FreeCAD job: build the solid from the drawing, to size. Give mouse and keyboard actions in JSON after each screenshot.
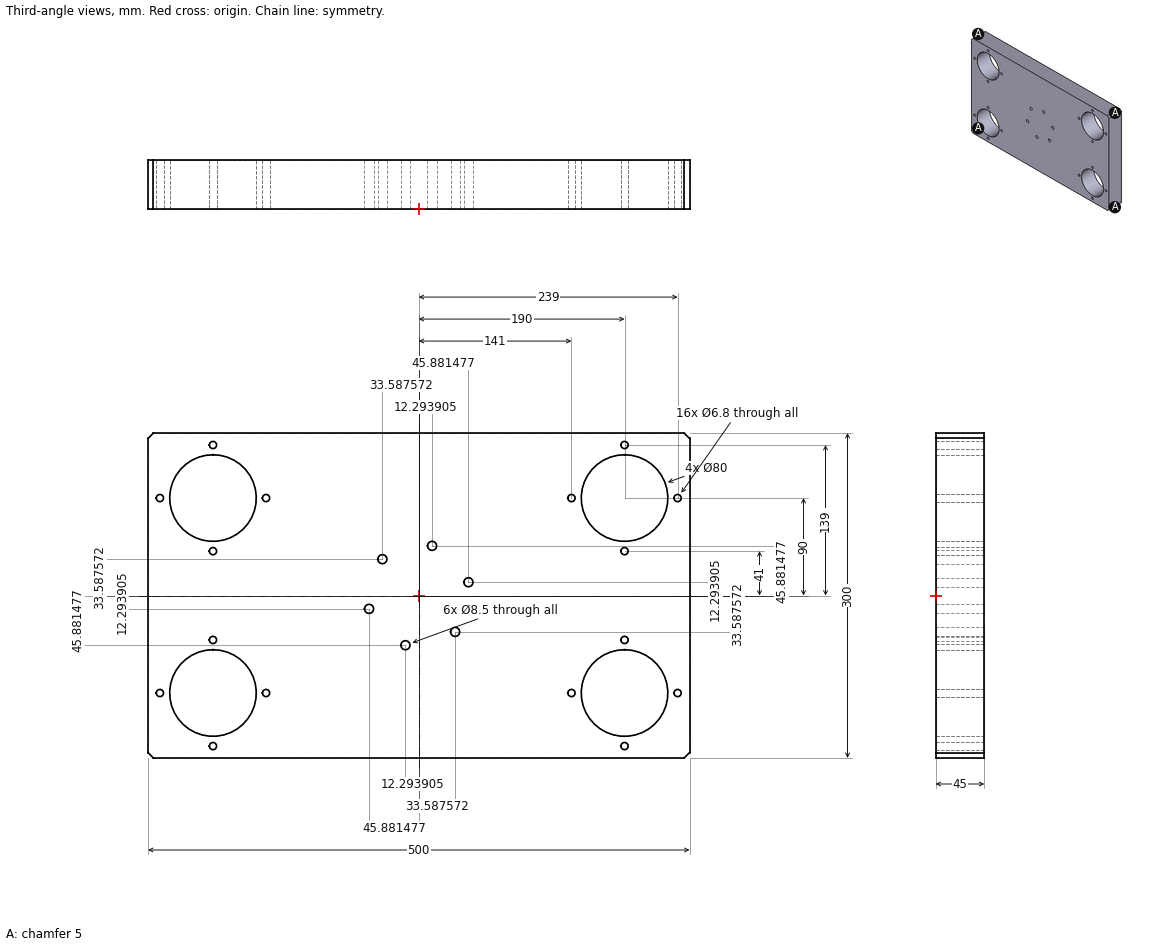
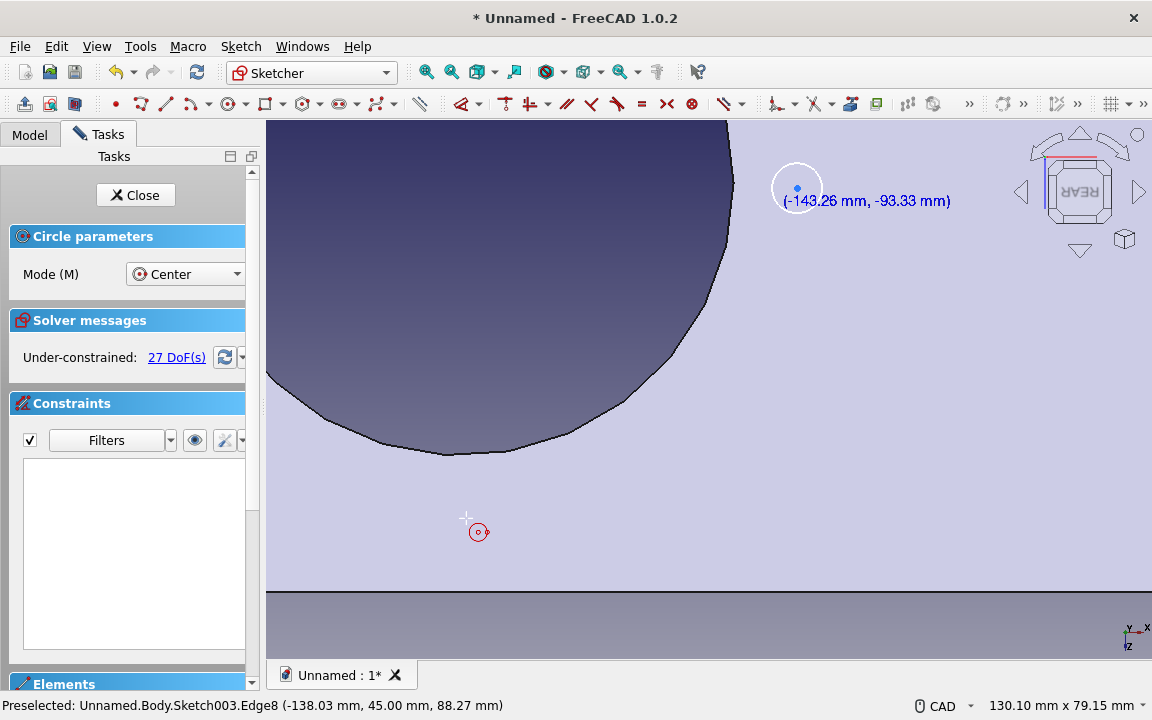
{"action": "scroll", "coordinate": [466, 518], "scroll_direction": "down", "scroll_amount": 10}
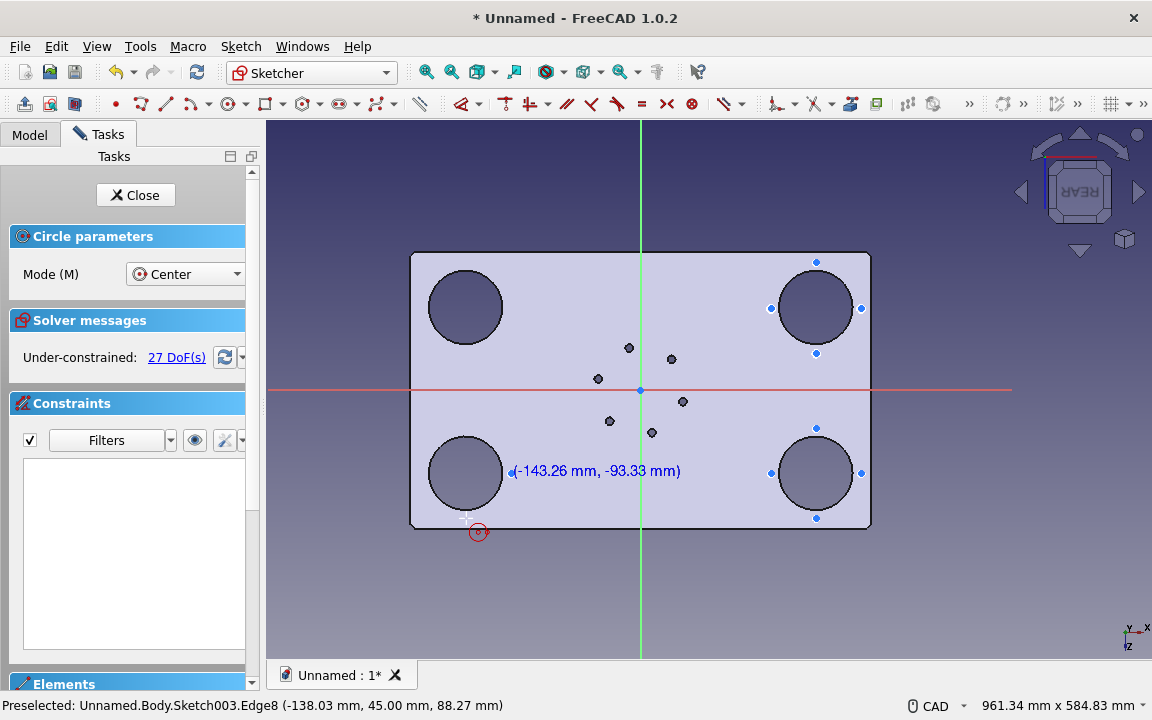
{"action": "left_click", "coordinate": [466, 518]}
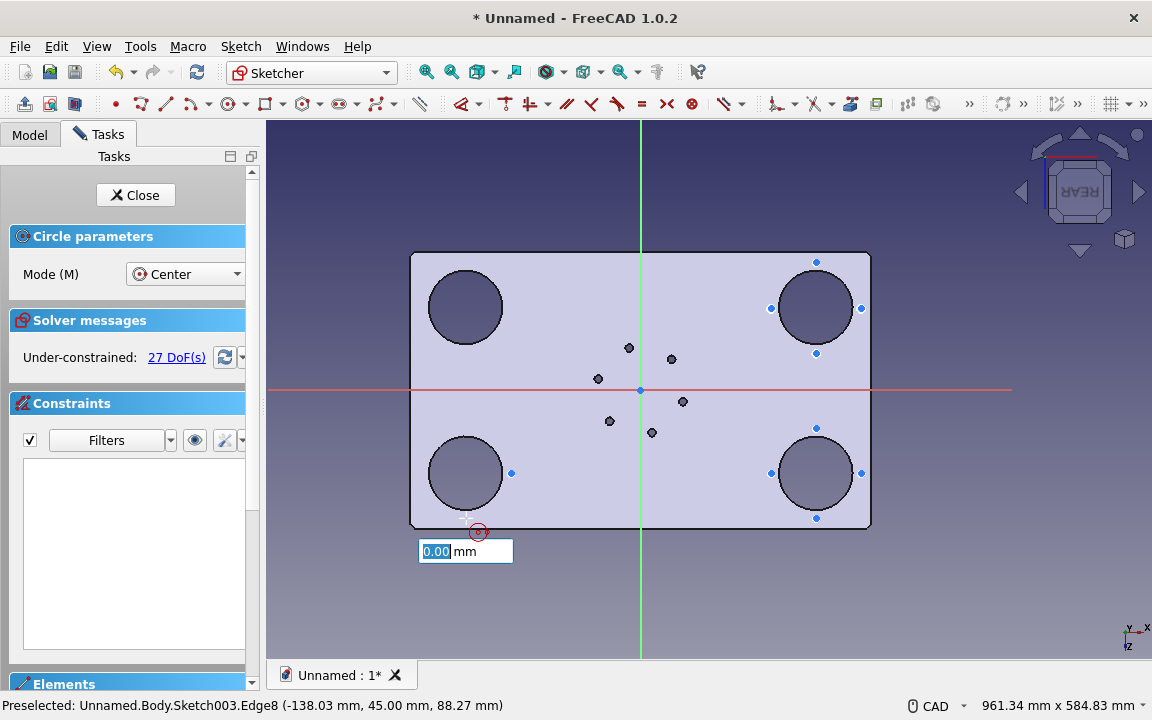
{"action": "scroll", "coordinate": [468, 516], "scroll_direction": "up", "scroll_amount": 9}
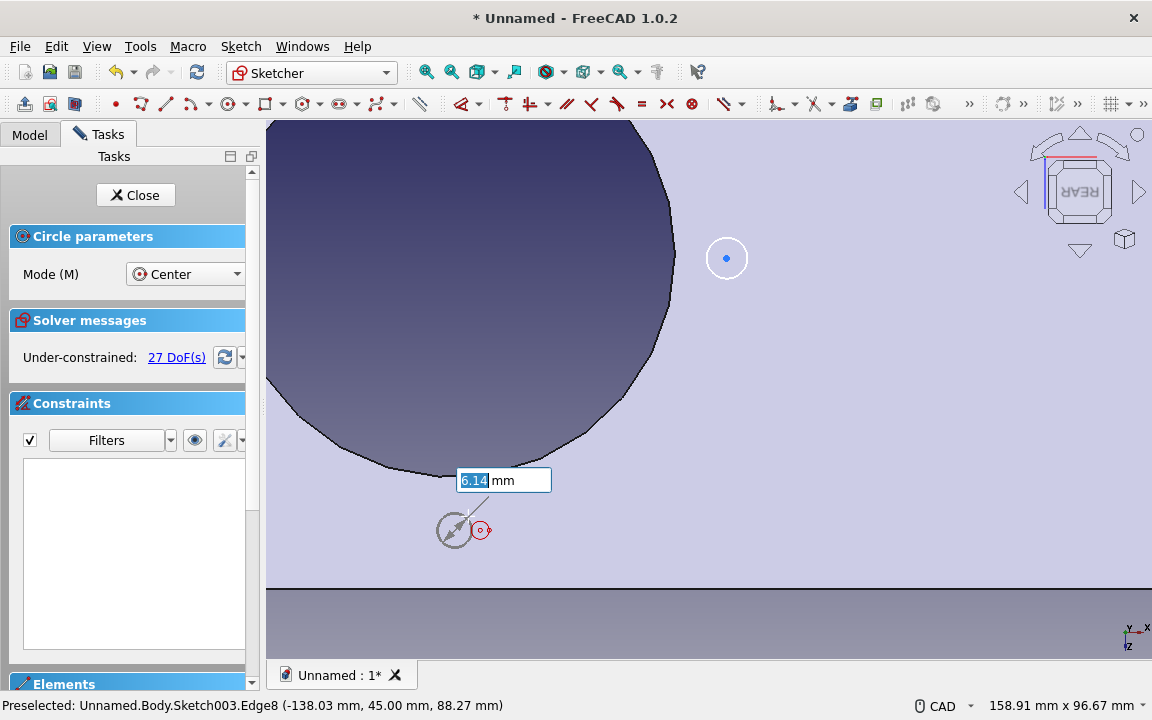
{"action": "left_click", "coordinate": [465, 514]}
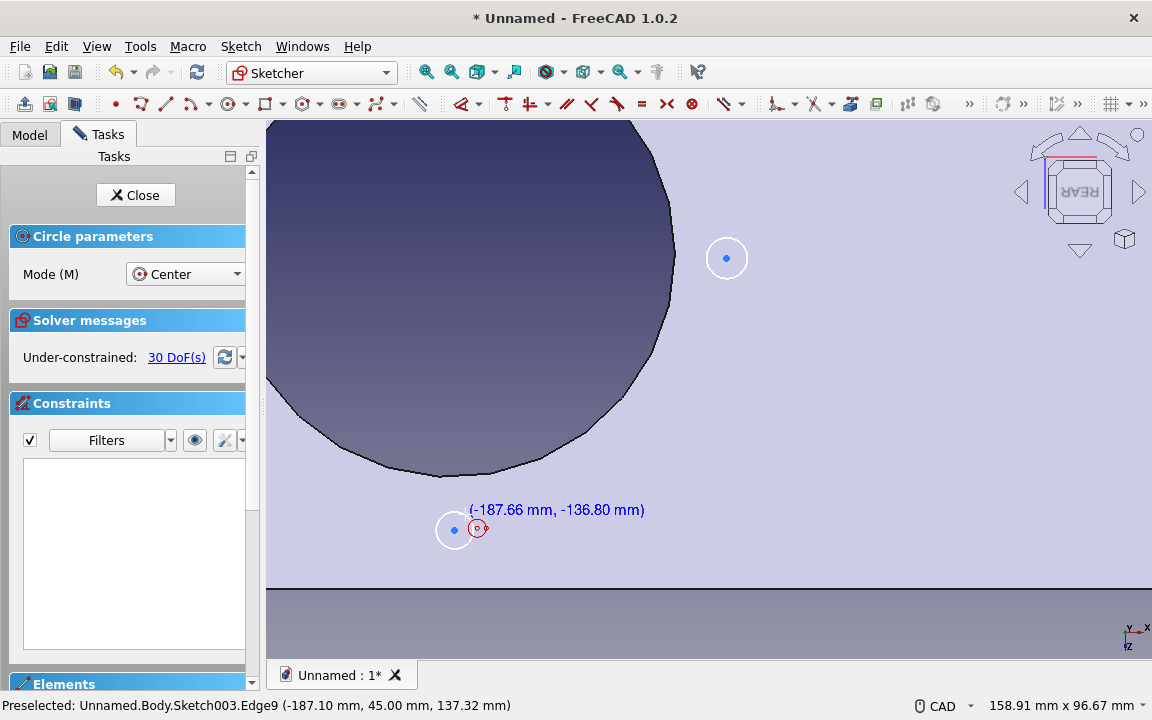
{"action": "scroll", "coordinate": [468, 516], "scroll_direction": "down", "scroll_amount": 9}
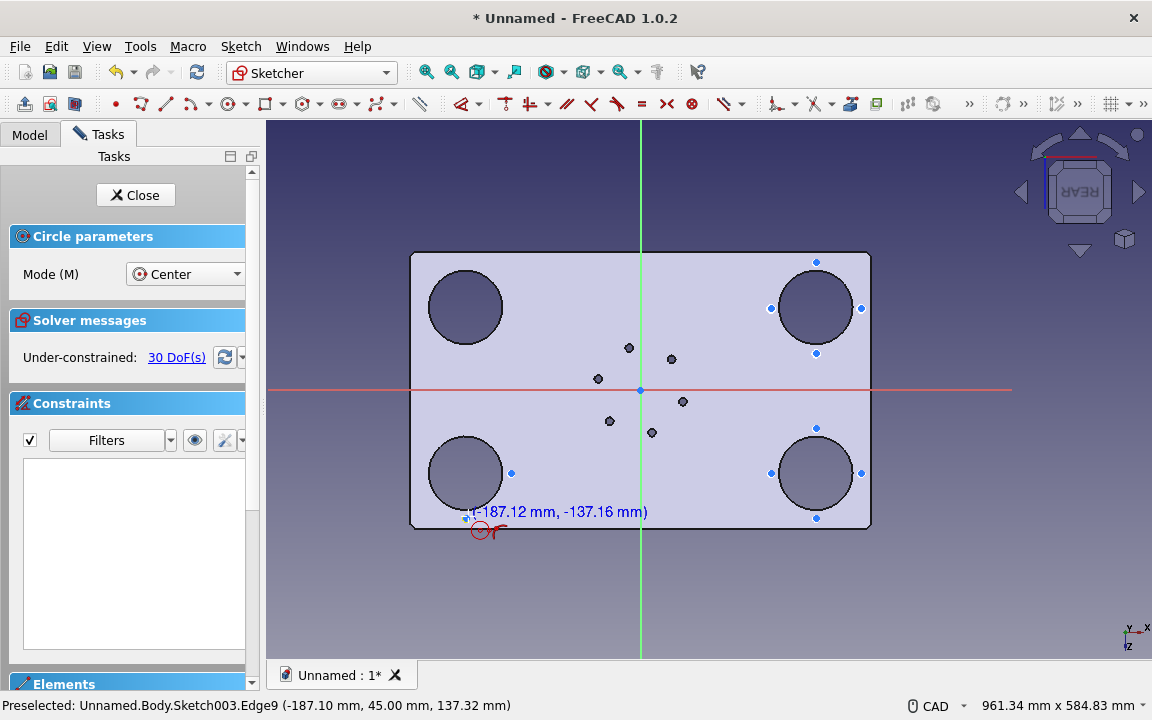
{"action": "scroll", "coordinate": [420, 473], "scroll_direction": "up", "scroll_amount": 10}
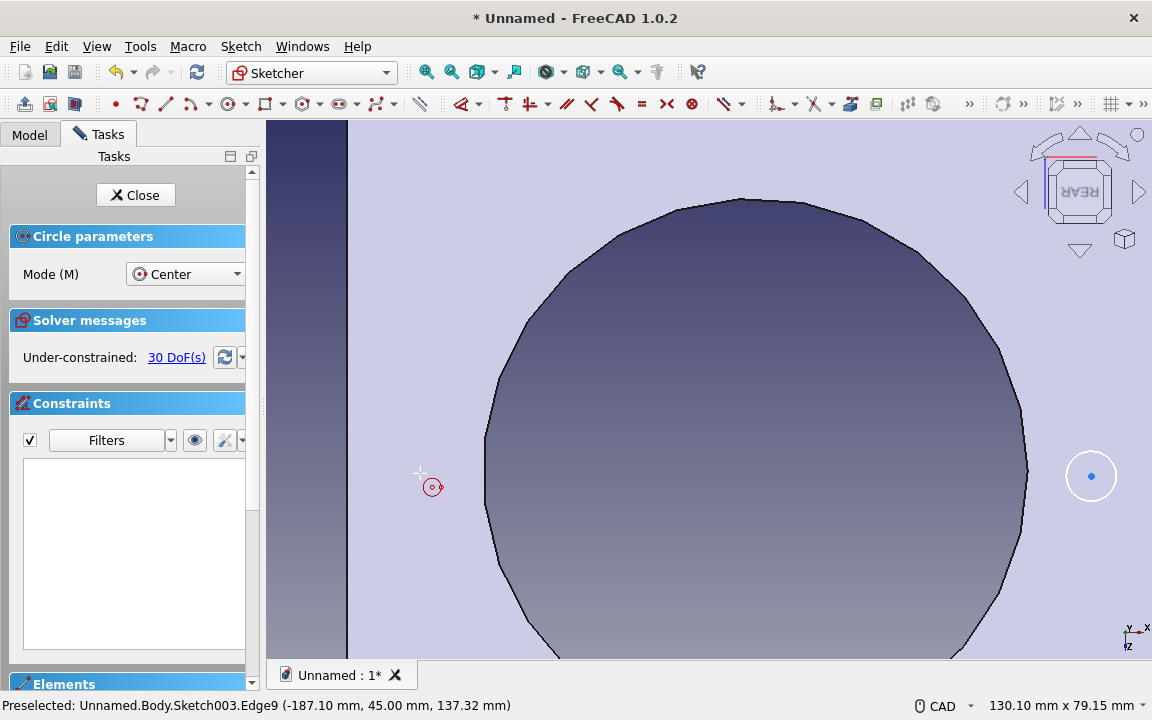
{"action": "scroll", "coordinate": [420, 473], "scroll_direction": "down", "scroll_amount": 10}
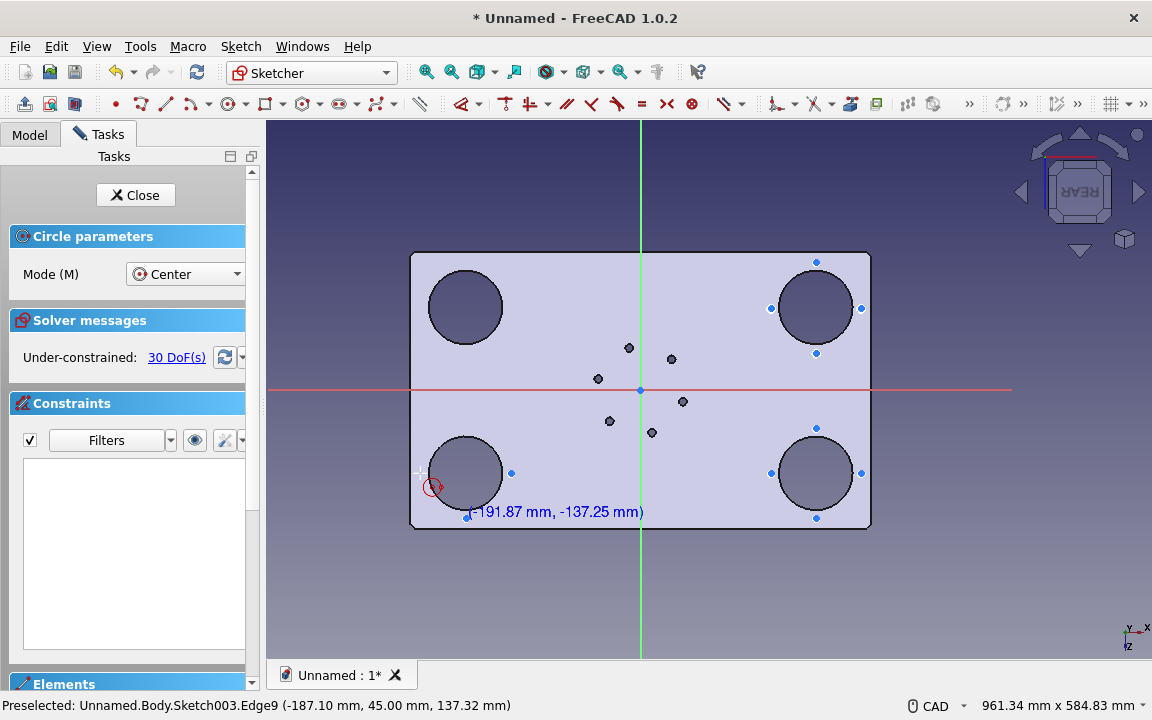
{"action": "left_click", "coordinate": [420, 473]}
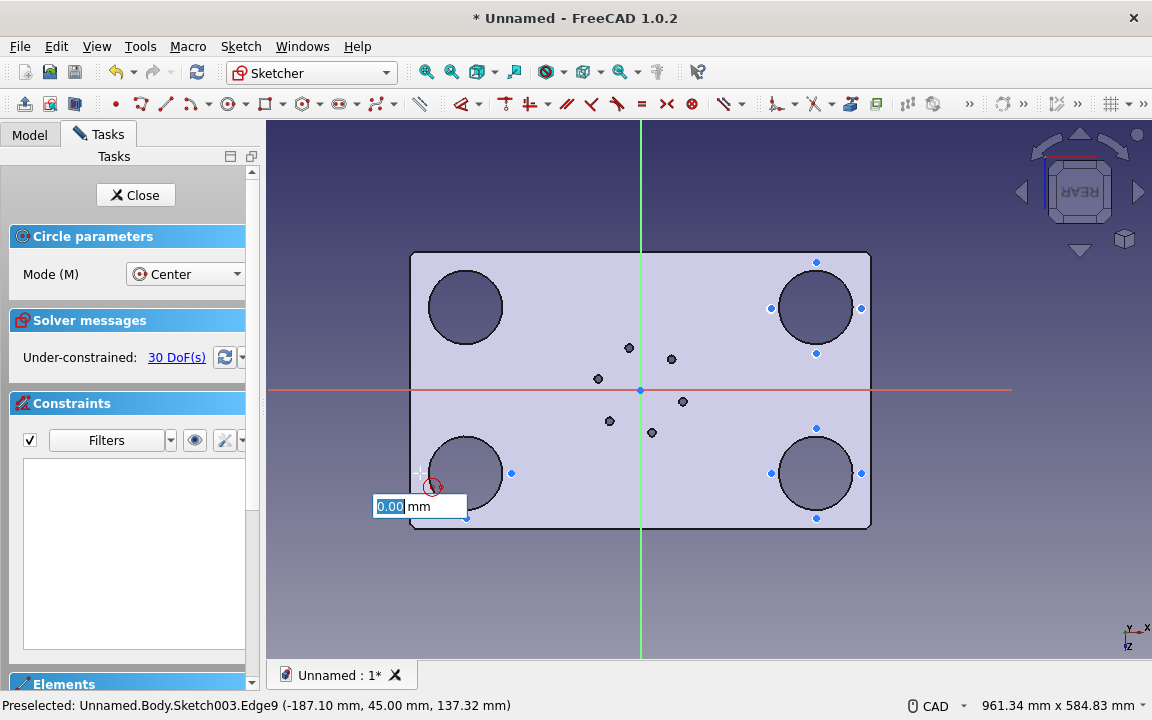
{"action": "scroll", "coordinate": [423, 471], "scroll_direction": "up", "scroll_amount": 9}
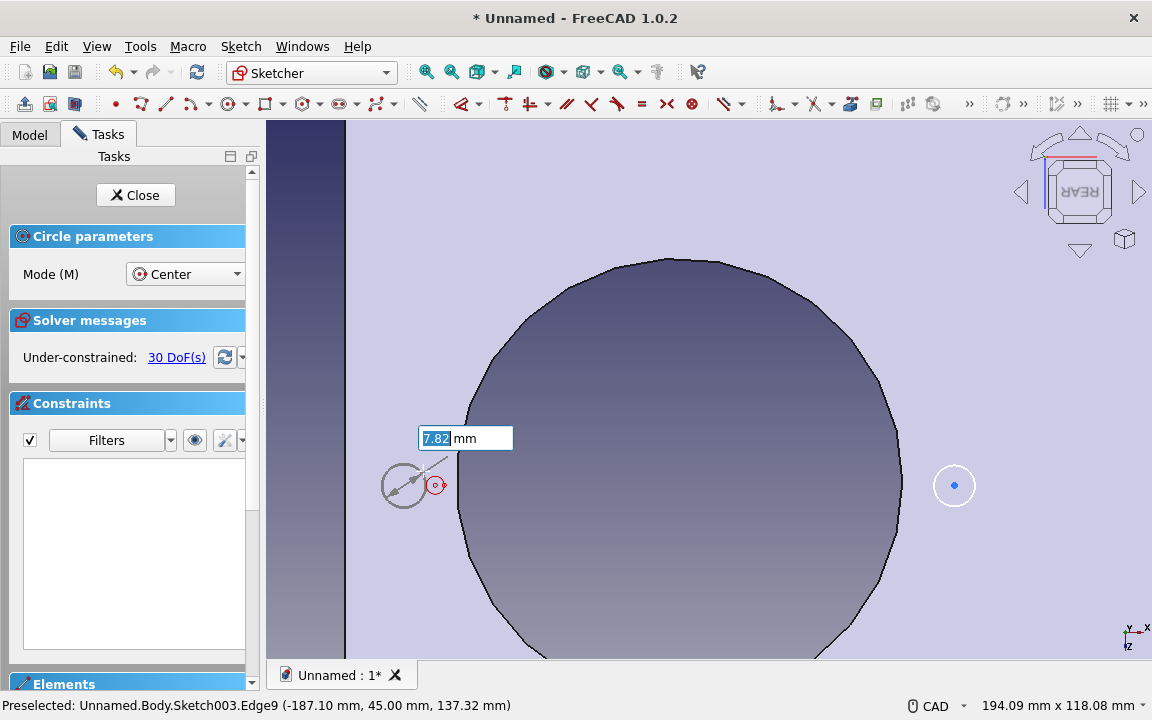
{"action": "left_click", "coordinate": [420, 468]}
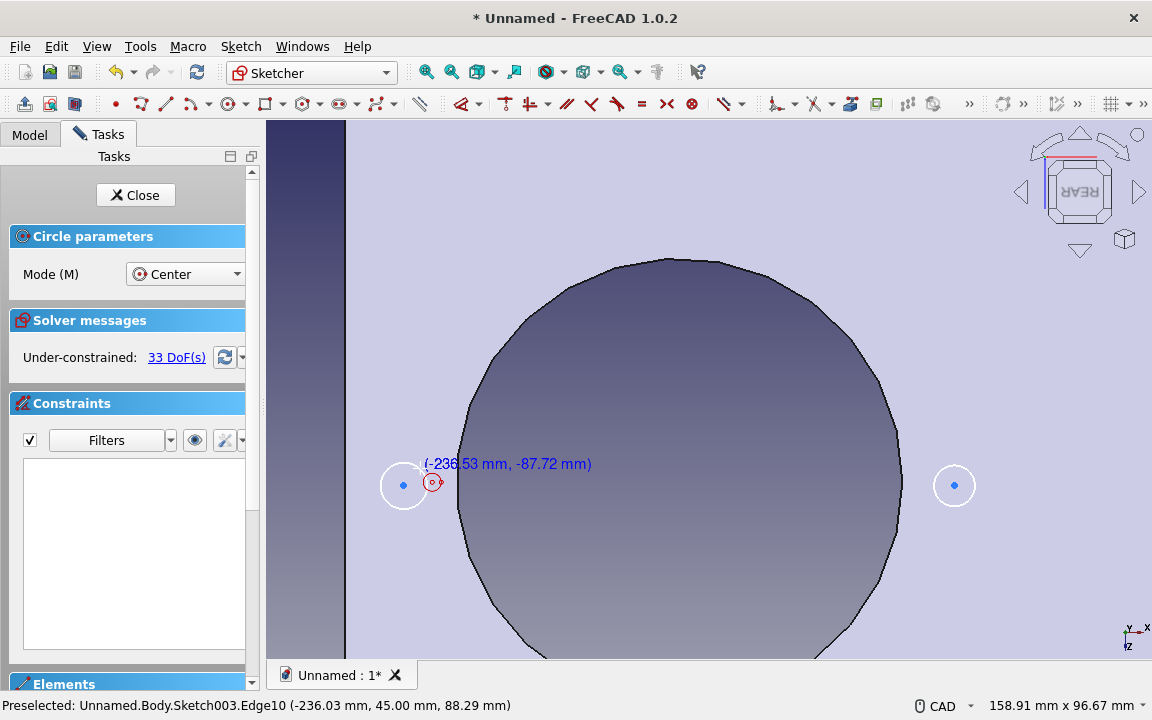
{"action": "scroll", "coordinate": [423, 471], "scroll_direction": "down", "scroll_amount": 9}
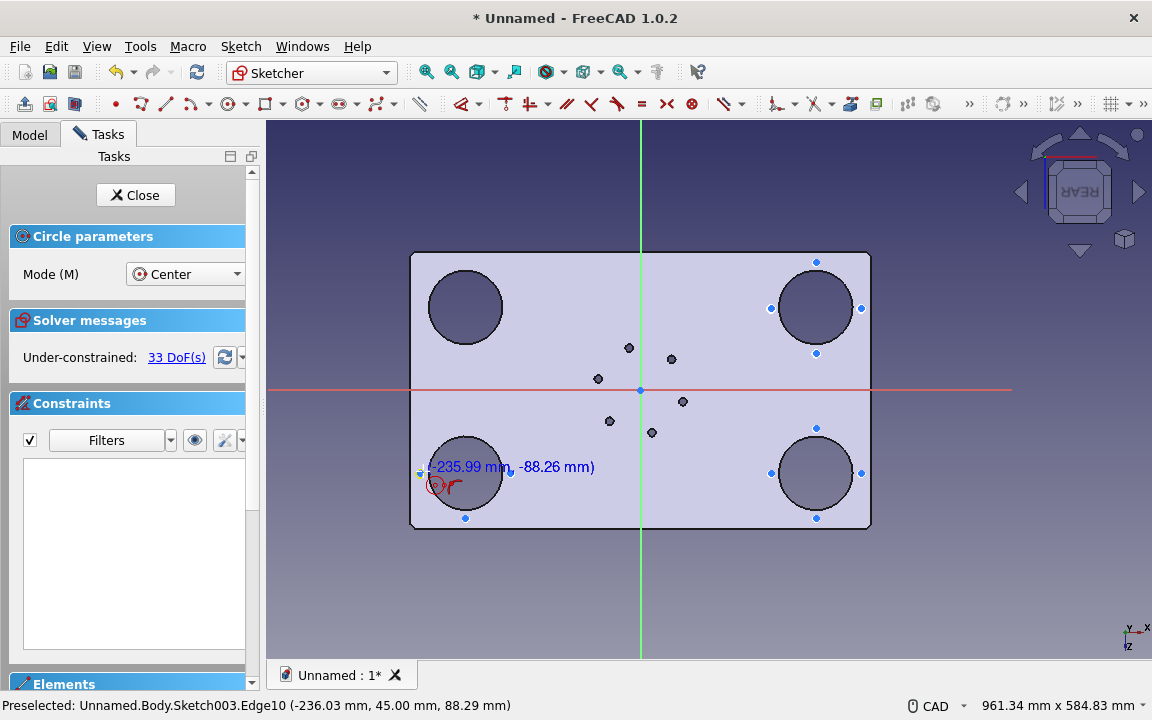
{"action": "left_click", "coordinate": [466, 428]}